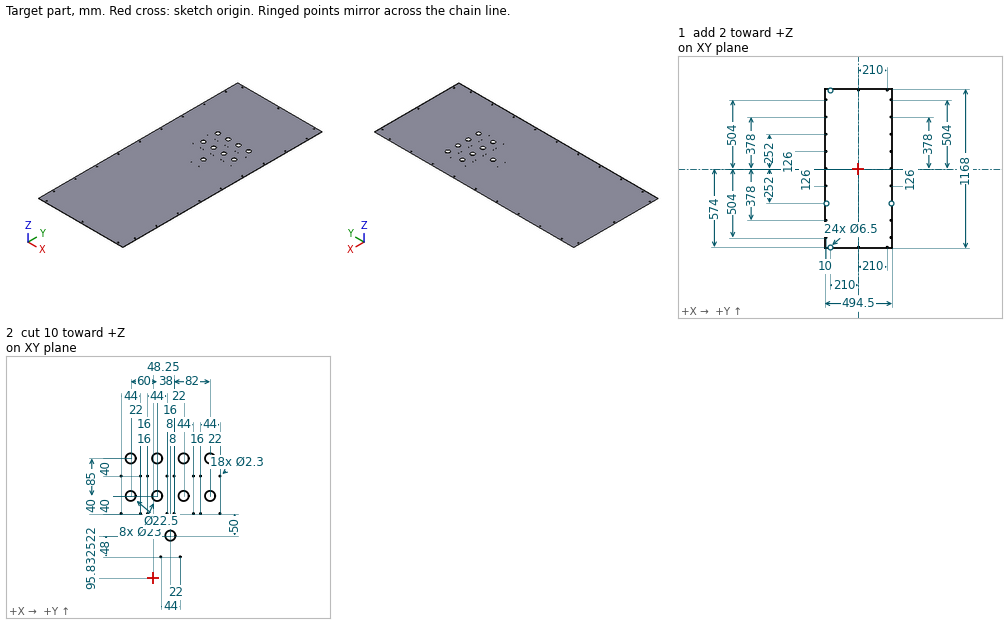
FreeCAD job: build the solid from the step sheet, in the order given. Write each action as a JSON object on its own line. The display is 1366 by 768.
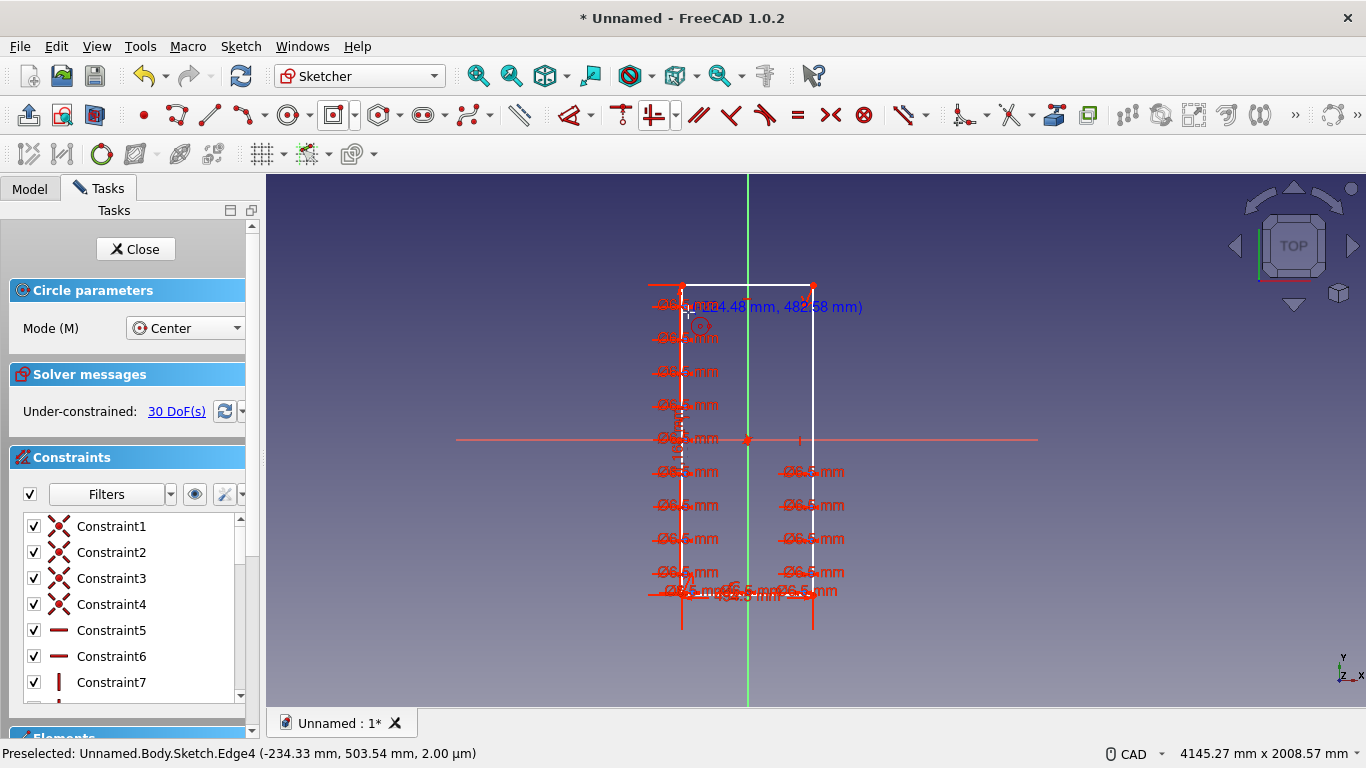
{"action": "scroll", "coordinate": [692, 288], "scroll_direction": "up", "scroll_amount": 17}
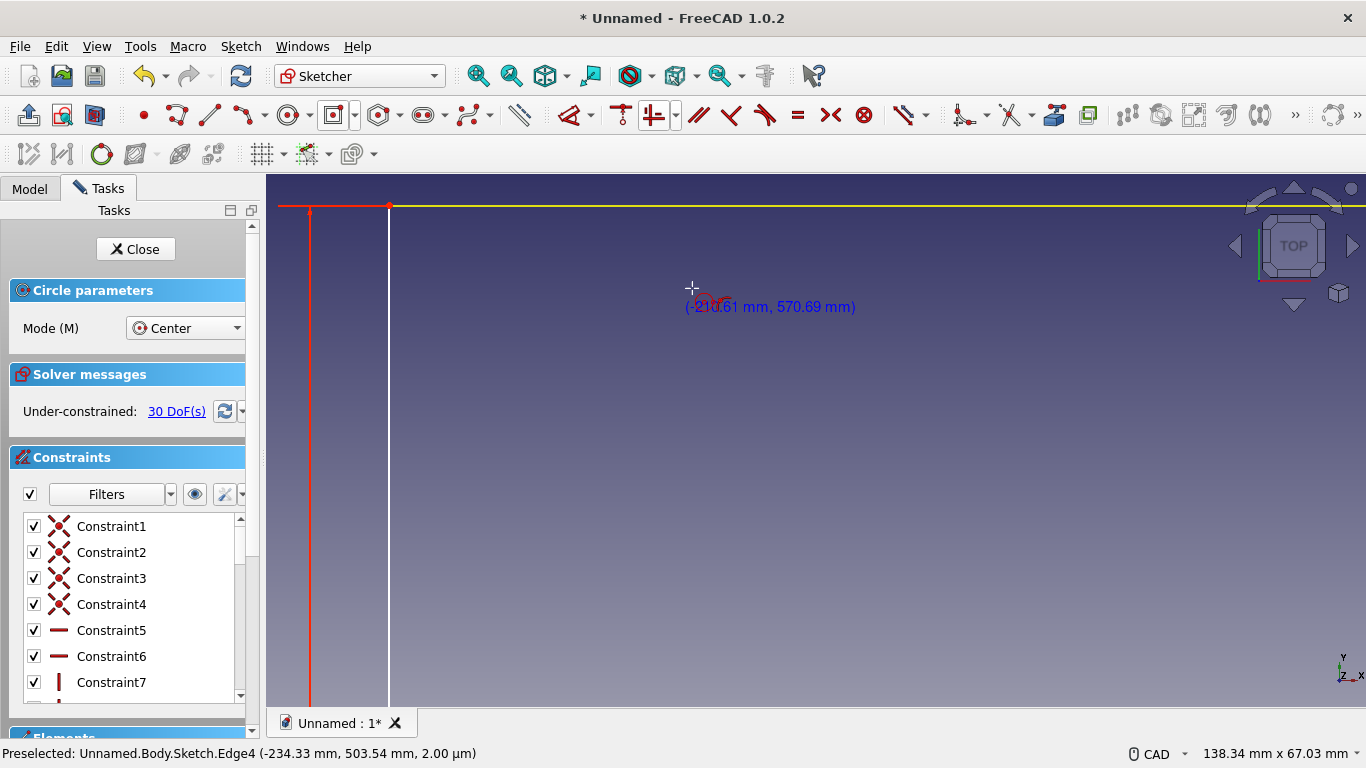
{"action": "scroll", "coordinate": [679, 253], "scroll_direction": "down", "scroll_amount": 16}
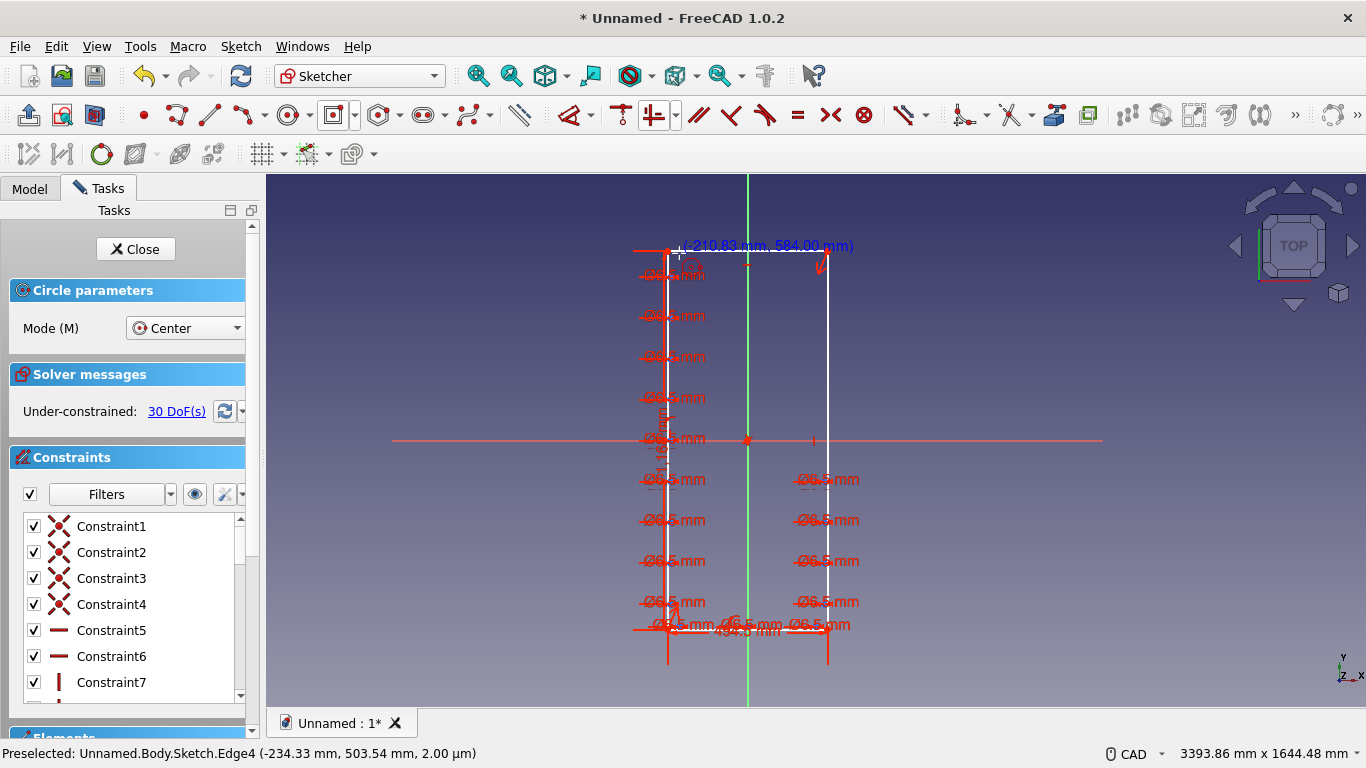
{"action": "scroll", "coordinate": [680, 254], "scroll_direction": "up", "scroll_amount": 8}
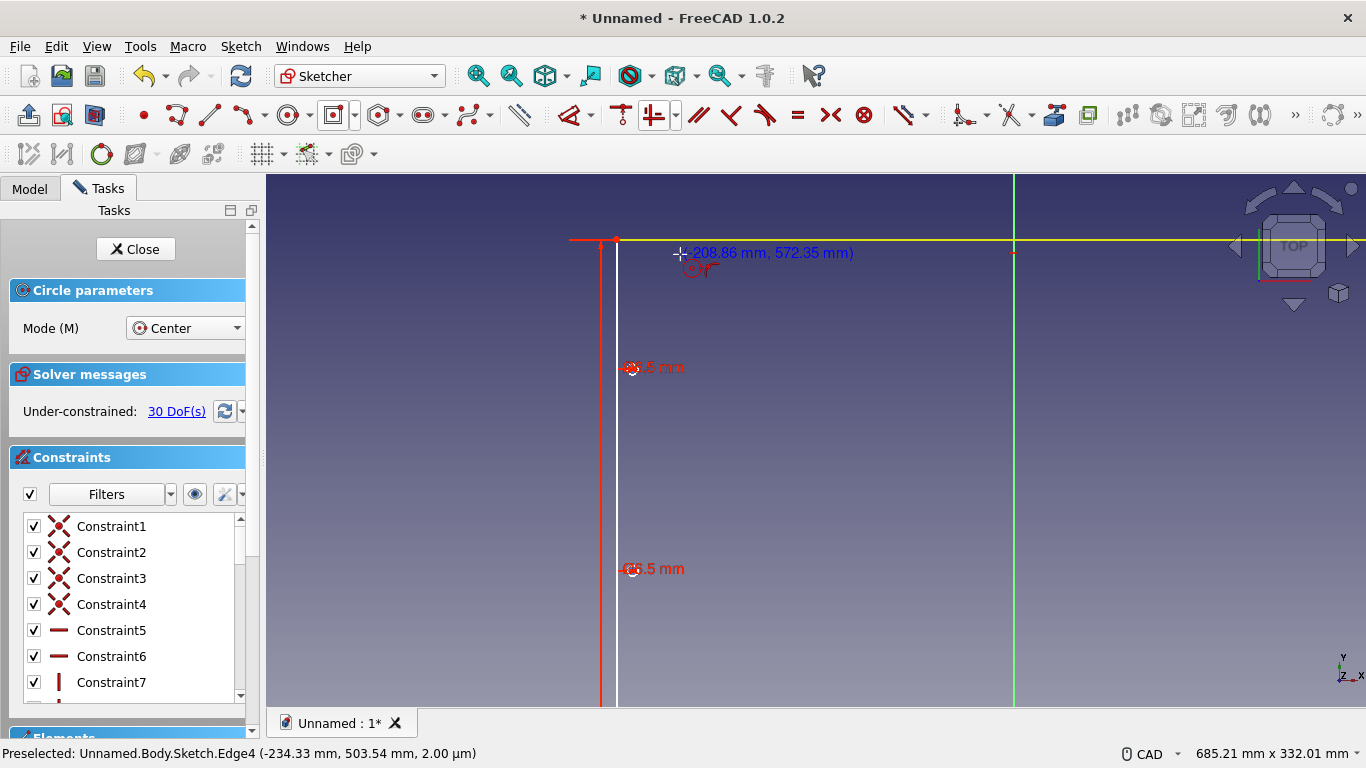
{"action": "left_click", "coordinate": [677, 256]}
{"action": "mouse_move", "coordinate": [680, 259]}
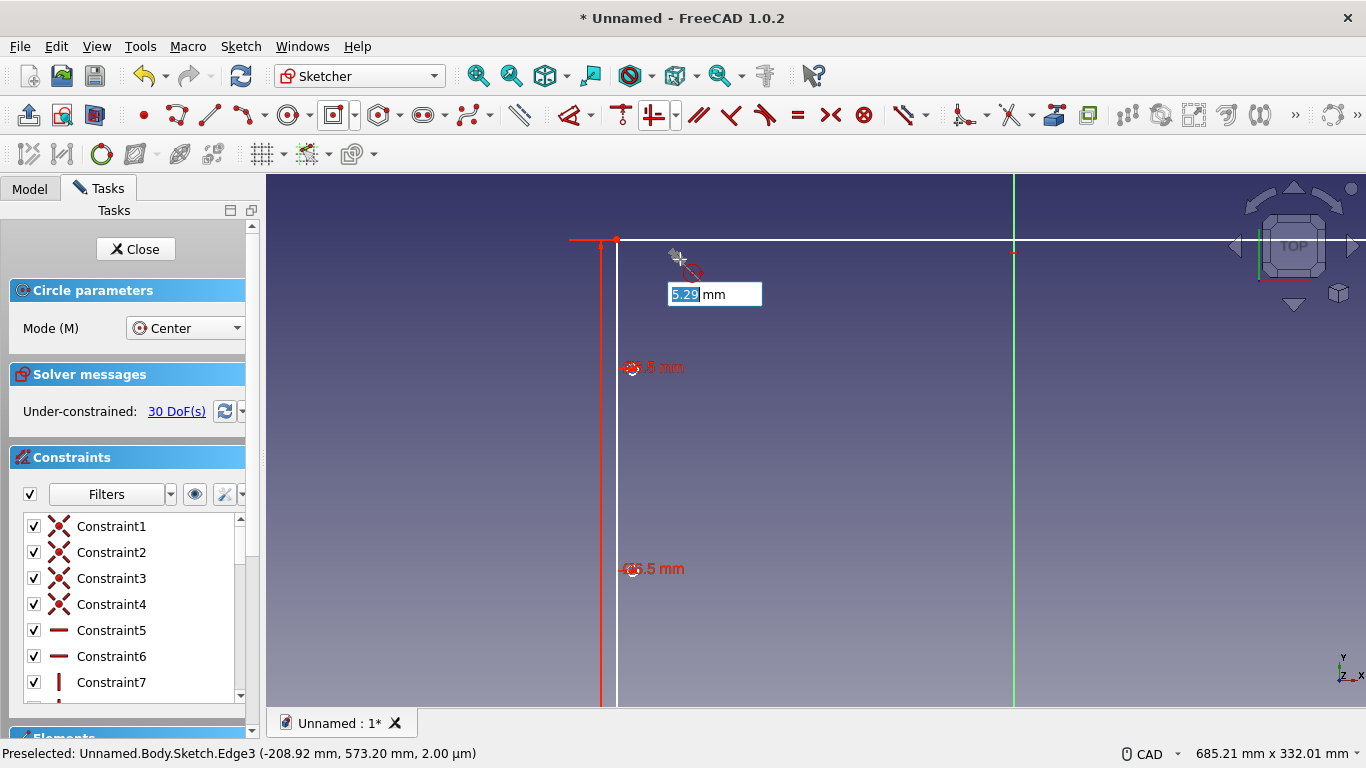
{"action": "type", "text": "6.5"}
{"action": "key", "text": "Return"}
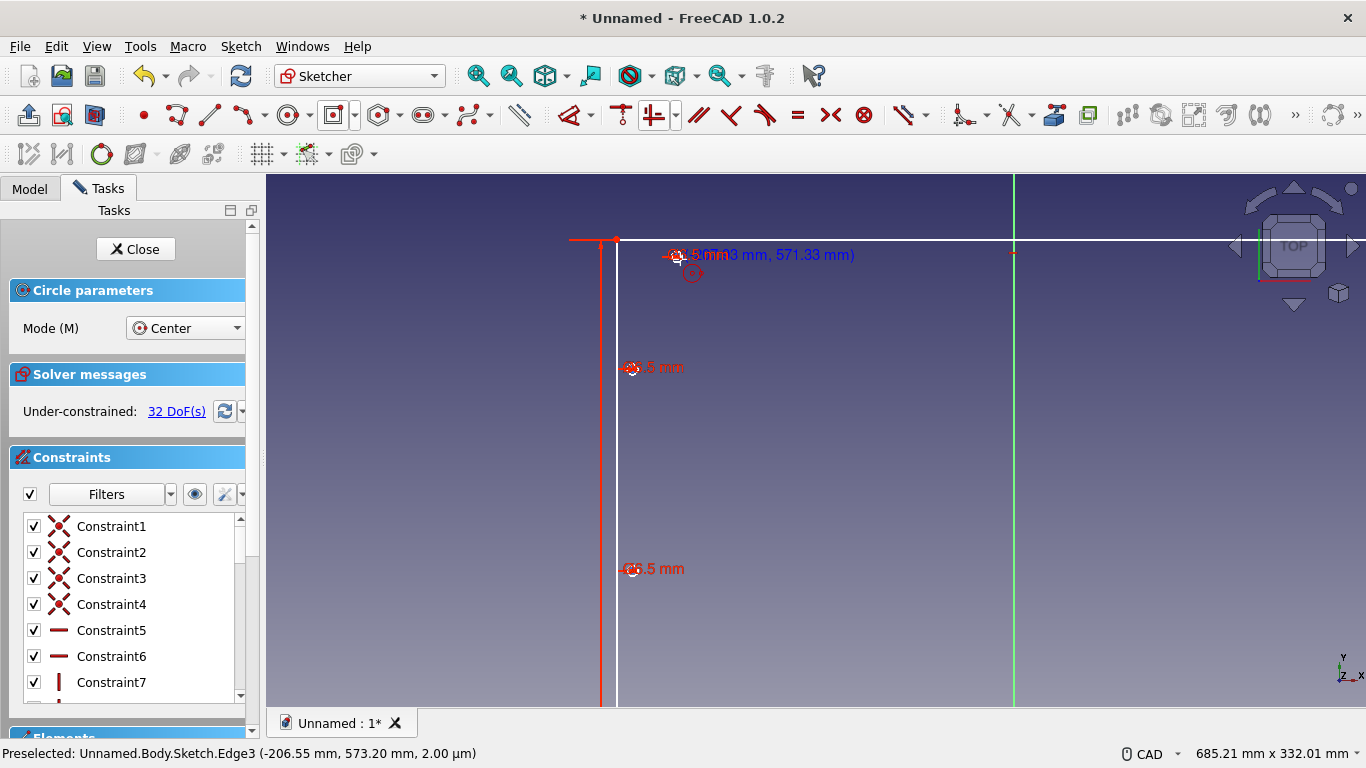
{"action": "scroll", "coordinate": [695, 295], "scroll_direction": "down", "scroll_amount": 9}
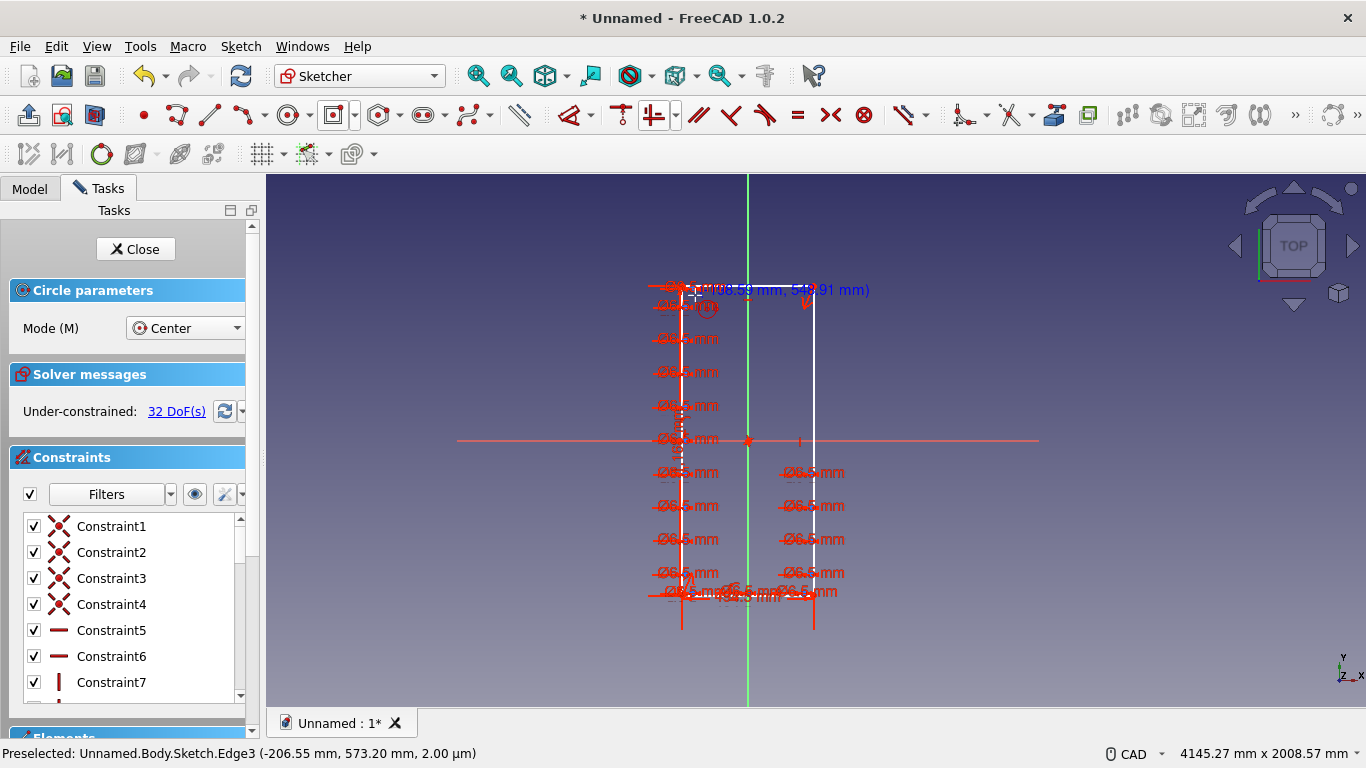
{"action": "scroll", "coordinate": [811, 441], "scroll_direction": "up", "scroll_amount": 17}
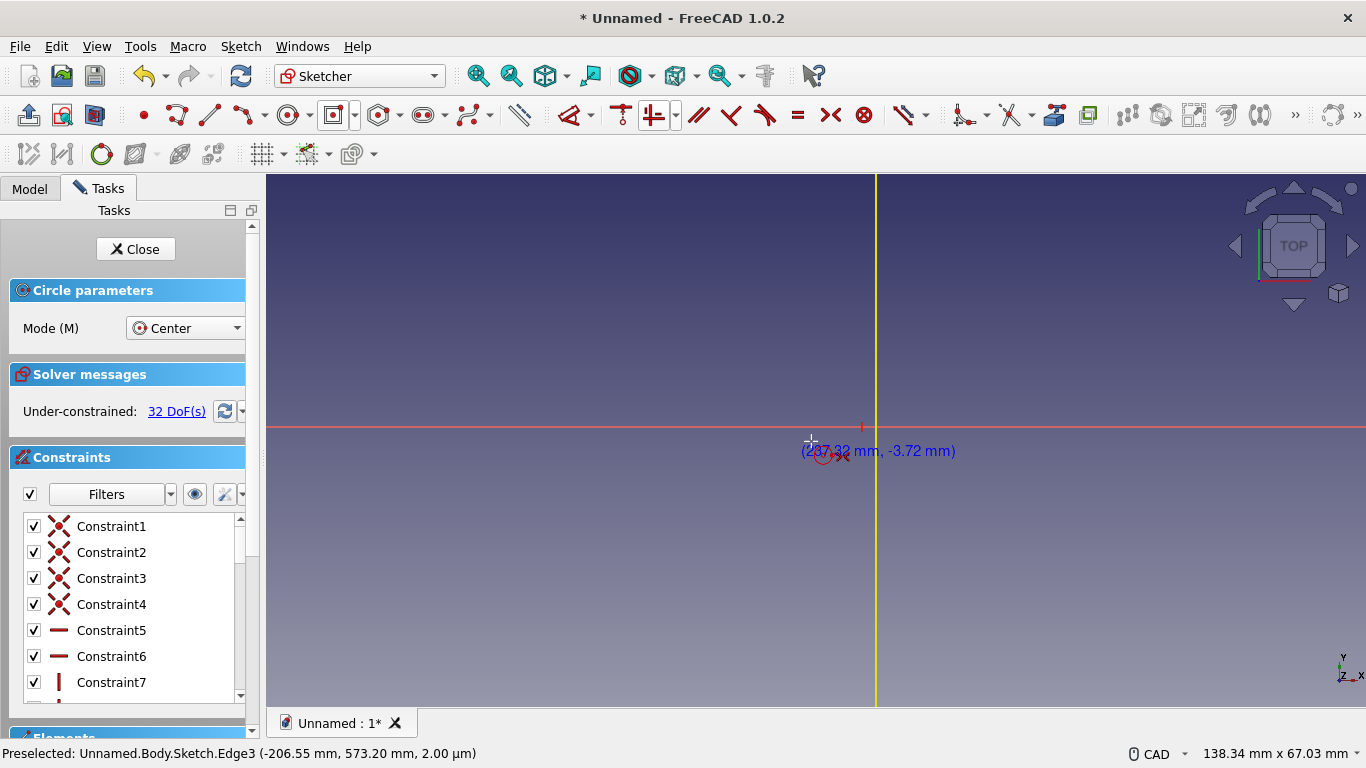
{"action": "scroll", "coordinate": [826, 441], "scroll_direction": "down", "scroll_amount": 16}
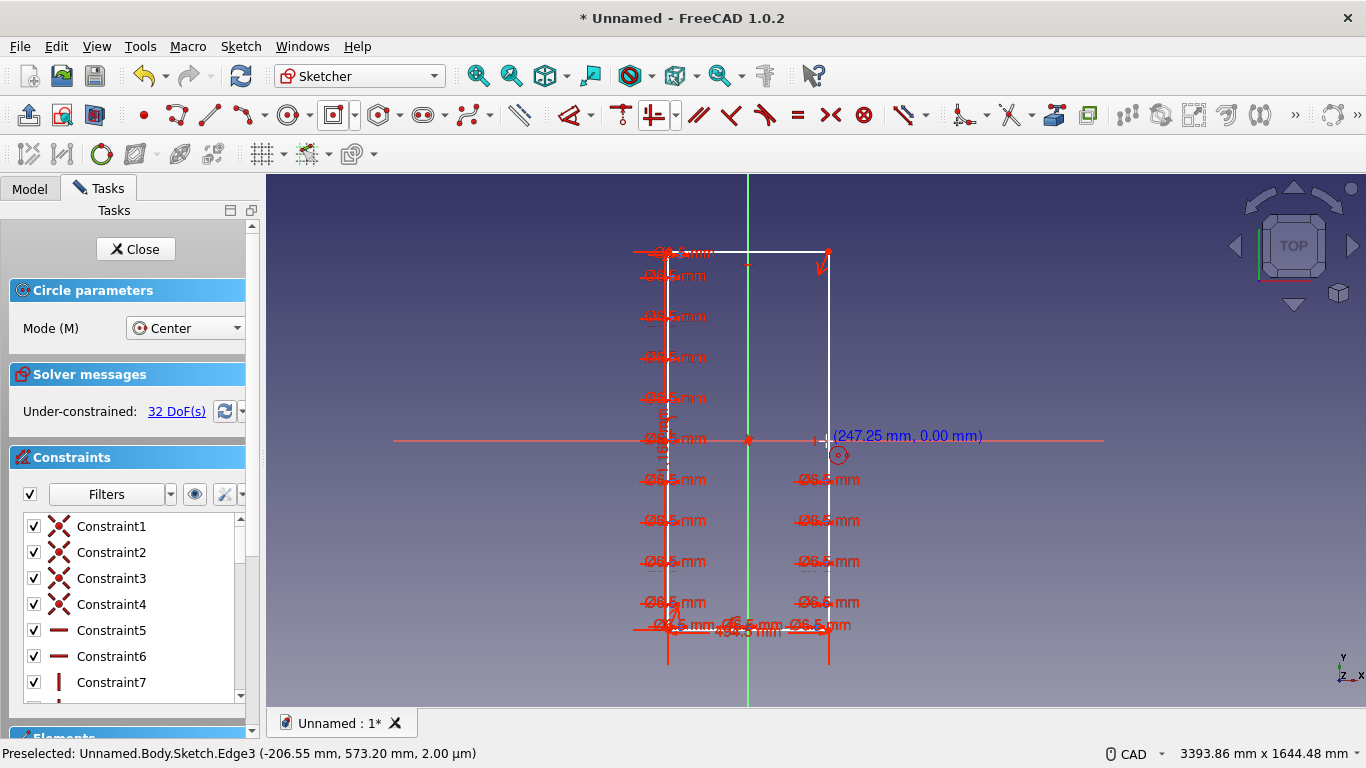
{"action": "scroll", "coordinate": [825, 441], "scroll_direction": "up", "scroll_amount": 8}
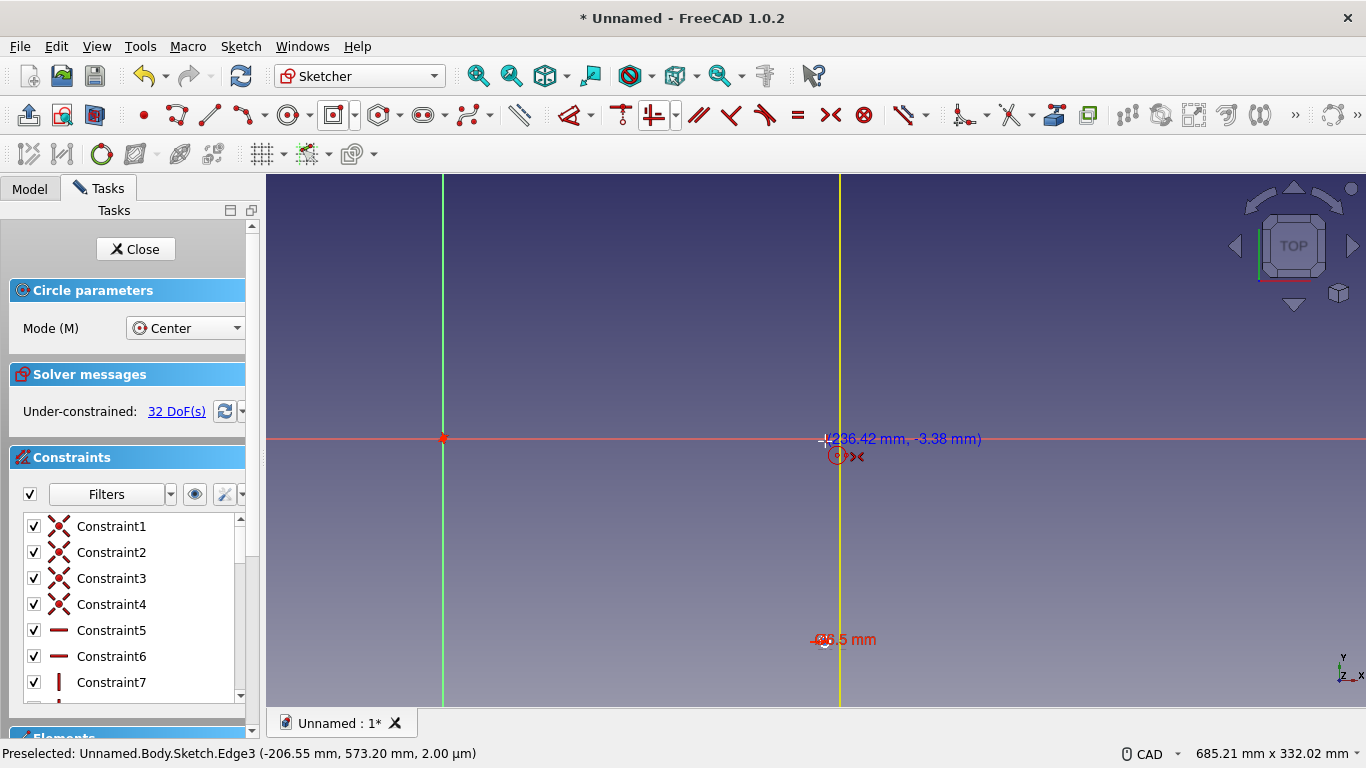
{"action": "left_click", "coordinate": [824, 439]}